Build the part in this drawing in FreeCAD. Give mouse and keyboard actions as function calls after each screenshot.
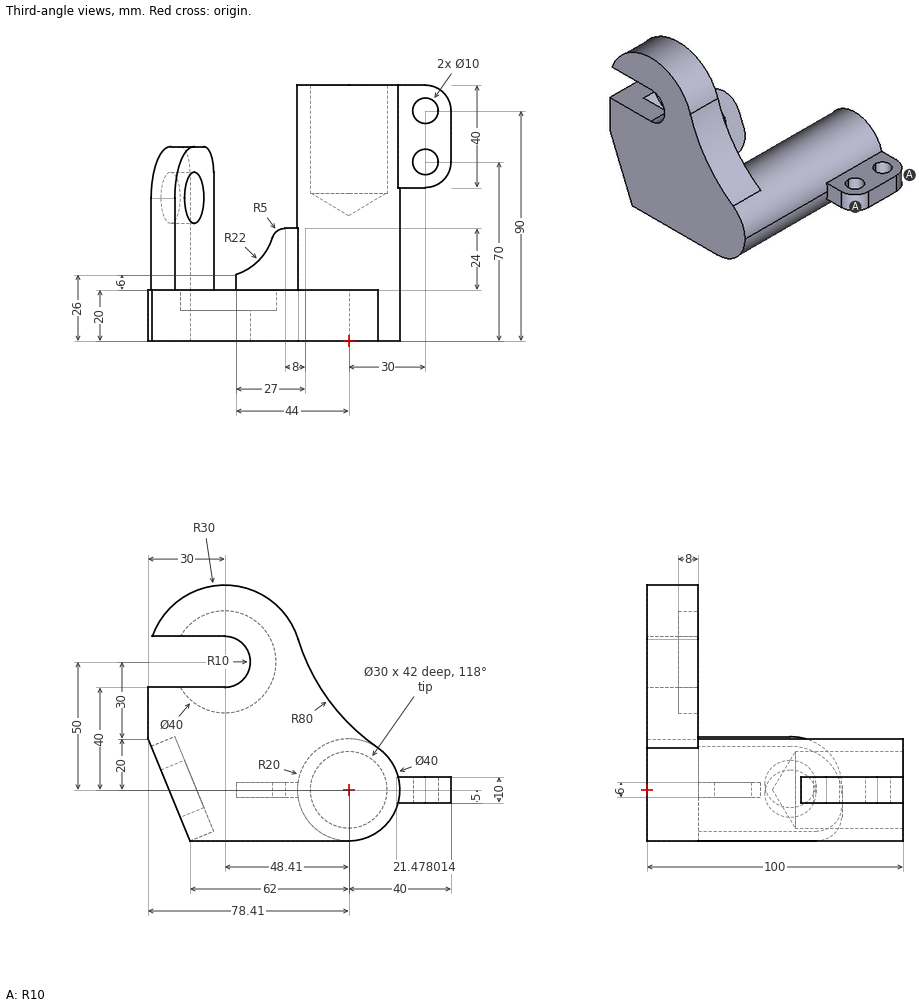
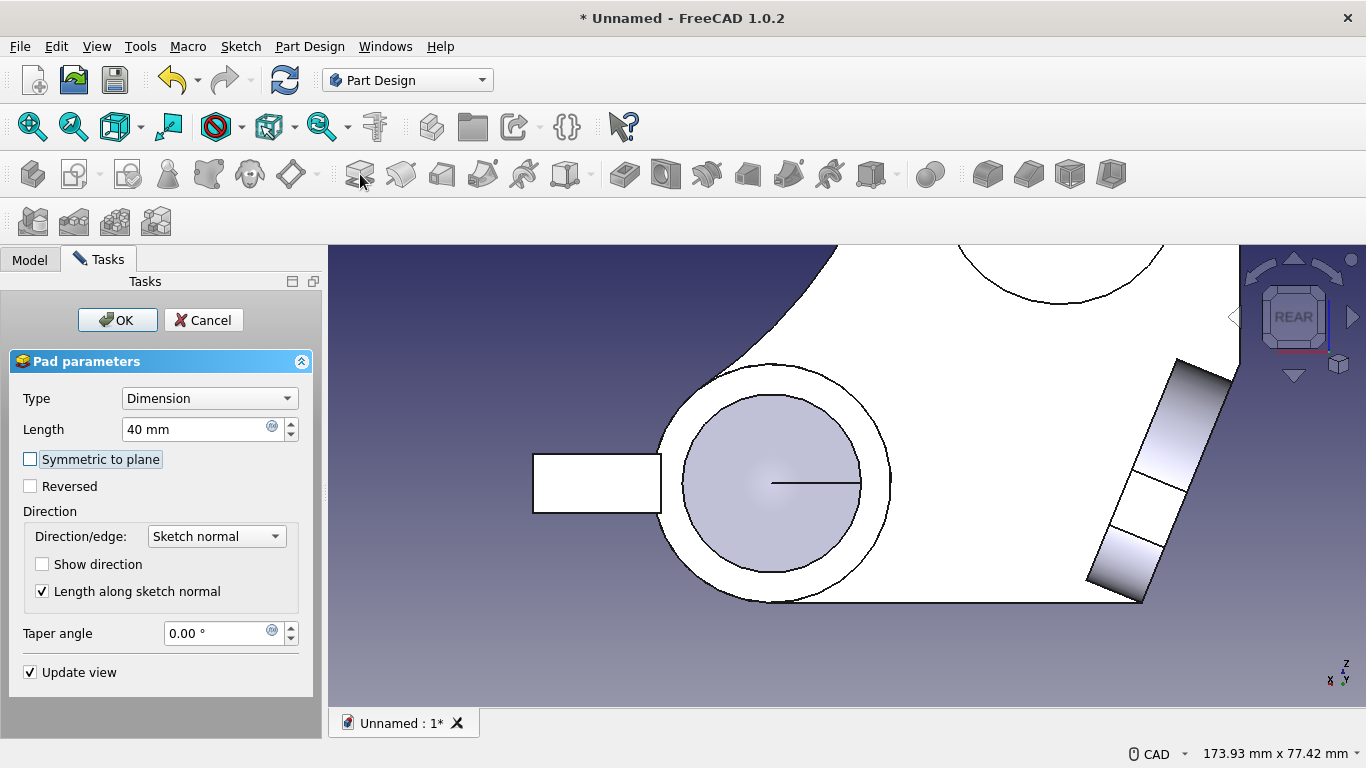
click(31, 486)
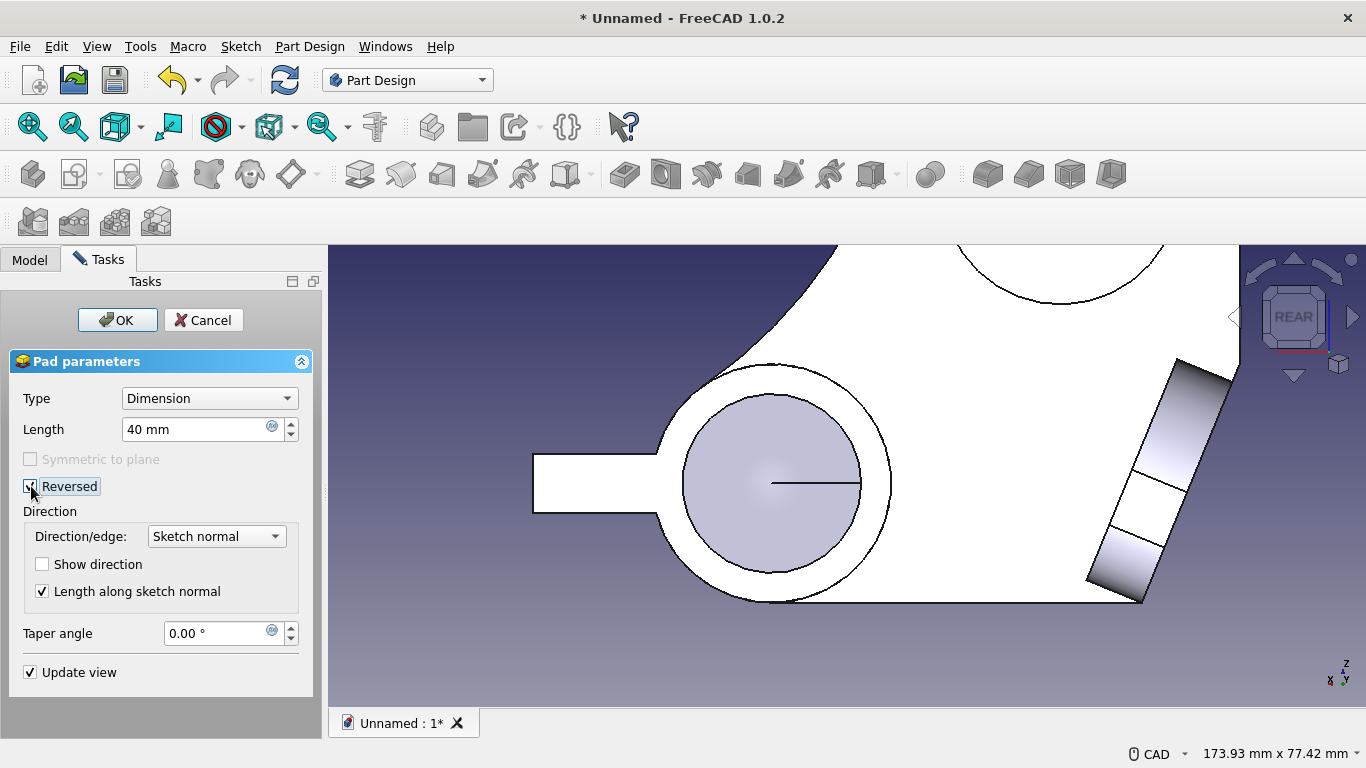
click(118, 320)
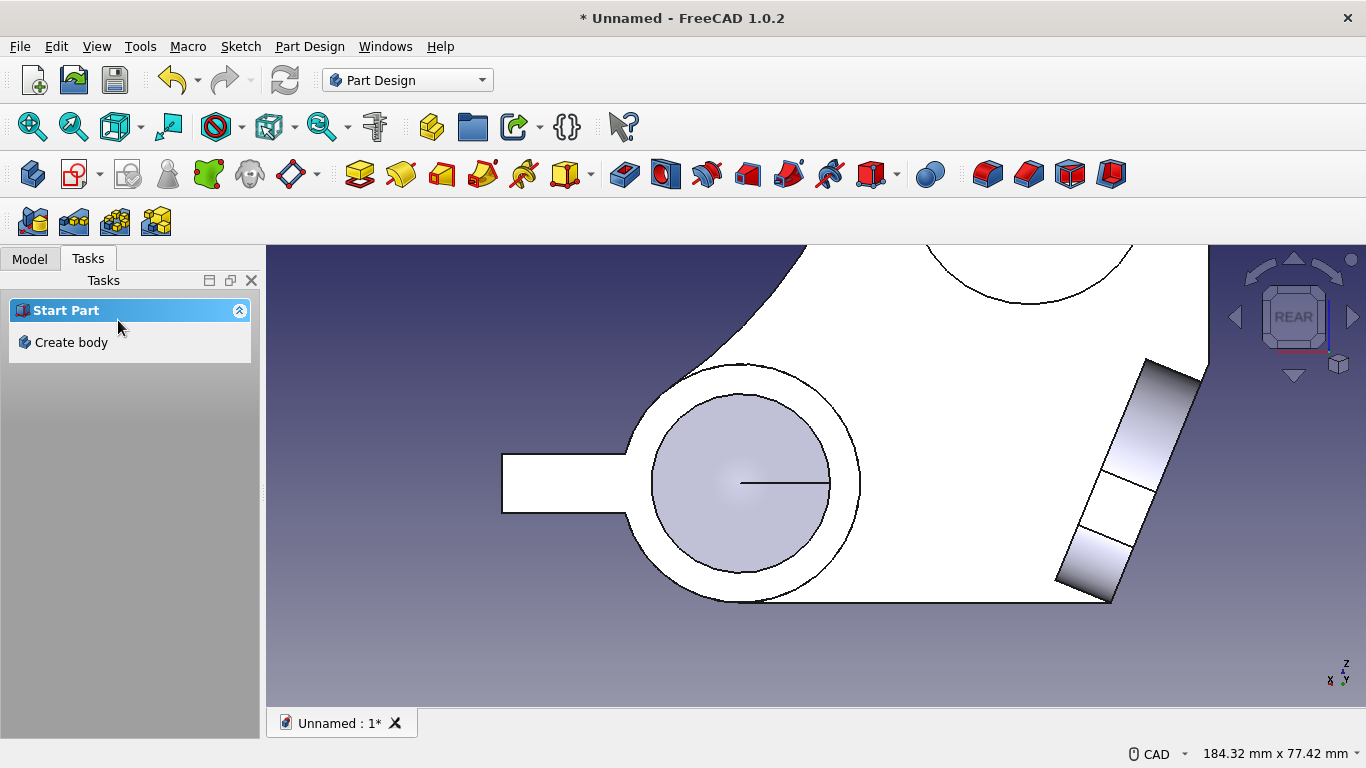
key(v)
key(f)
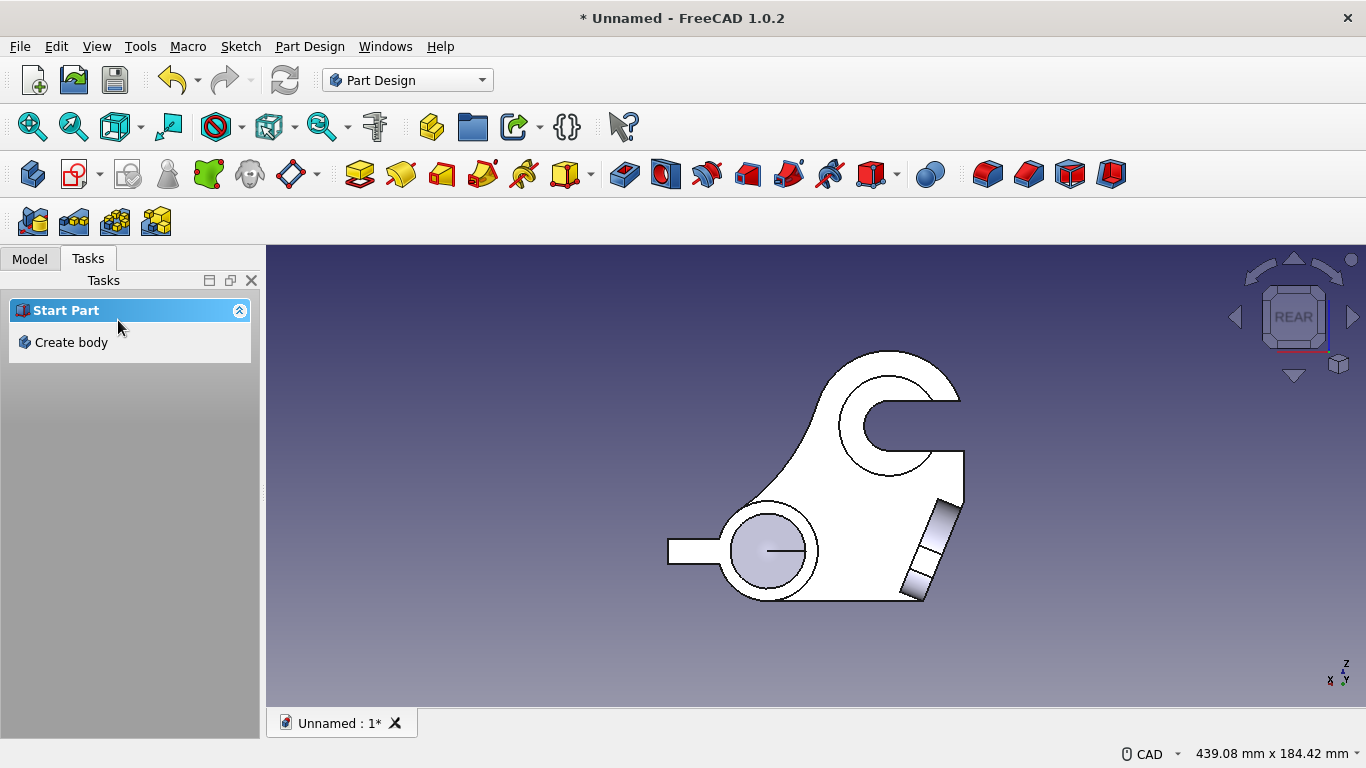
key(0)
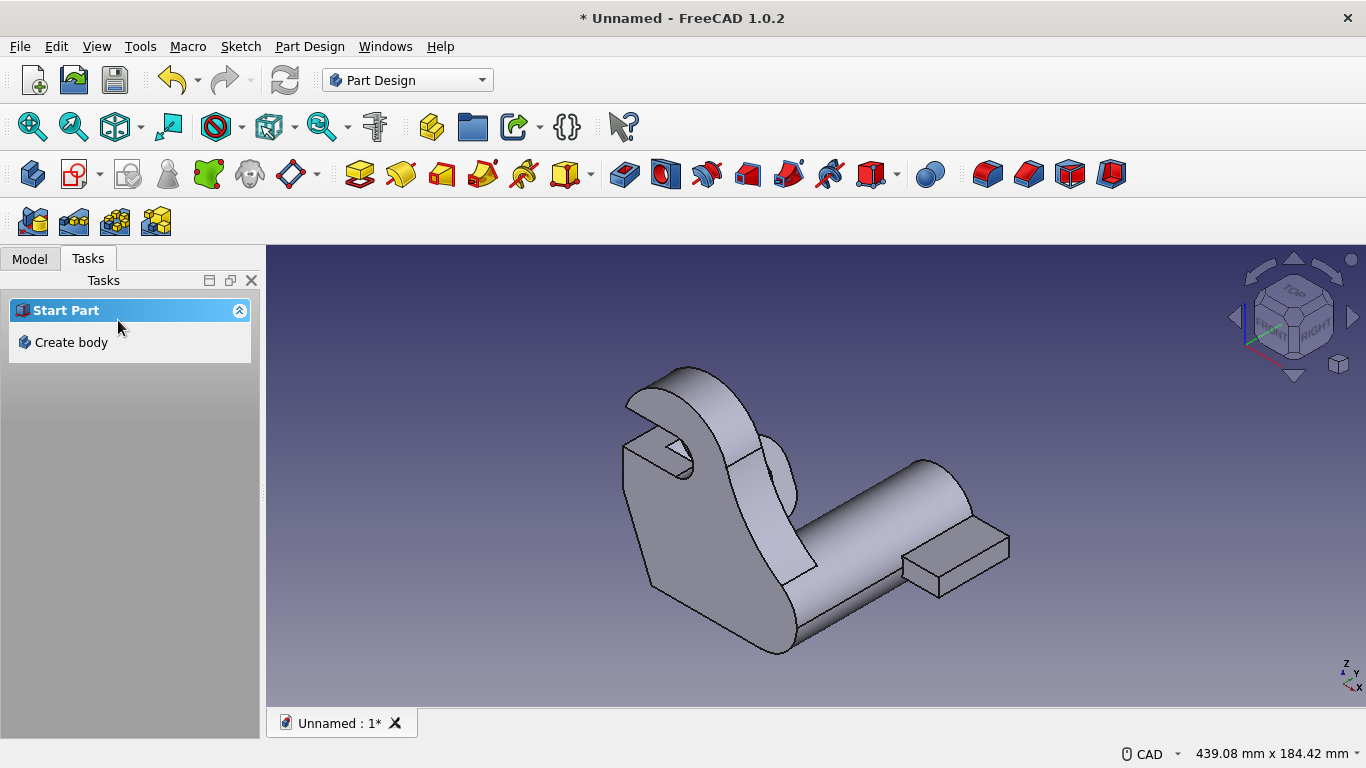
click(939, 587)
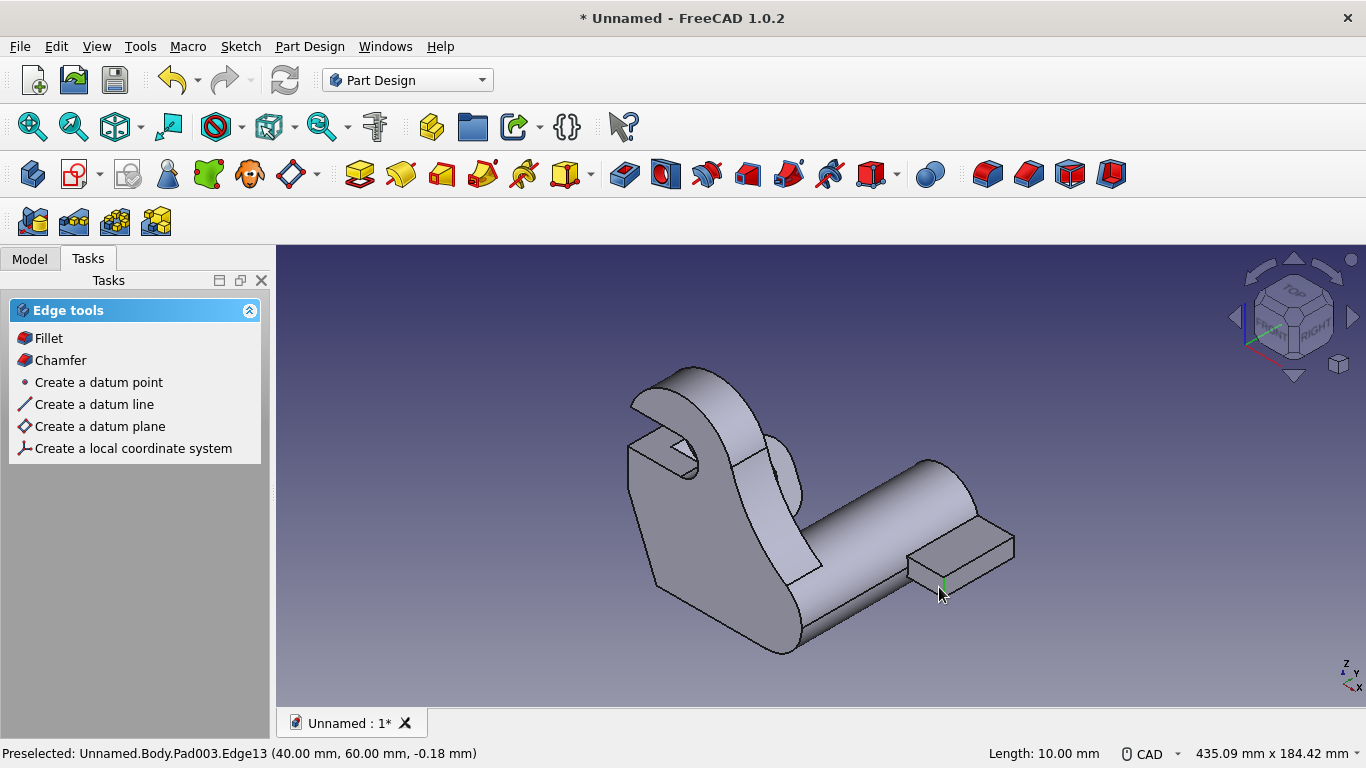
key(2)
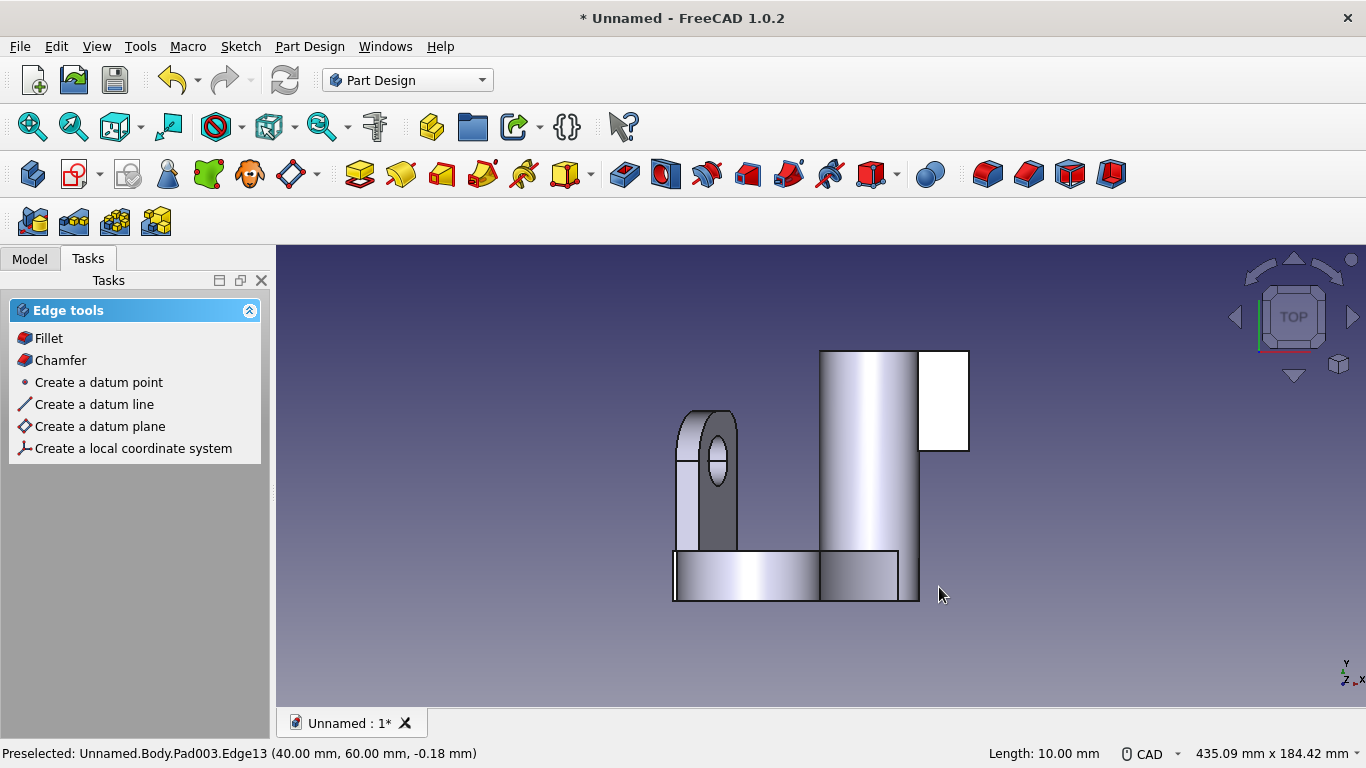
key(1)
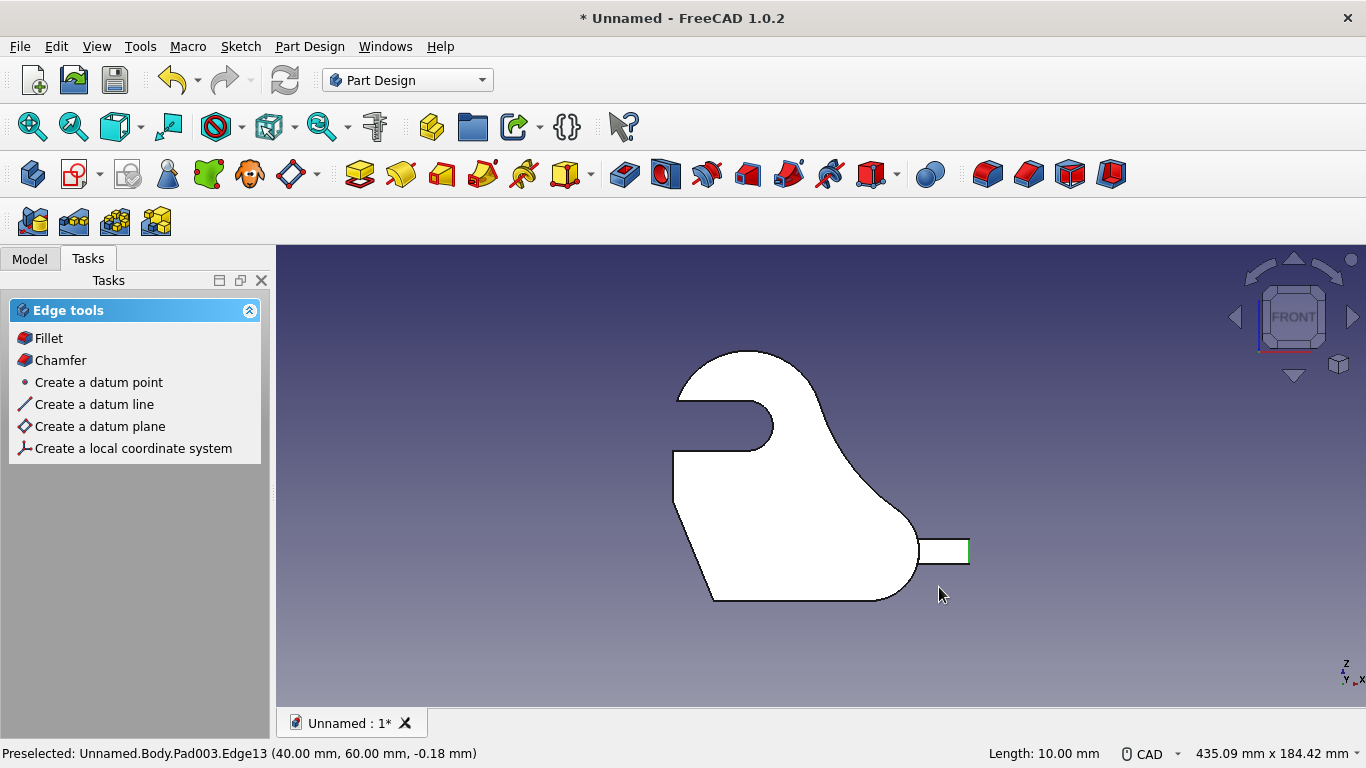
key(3)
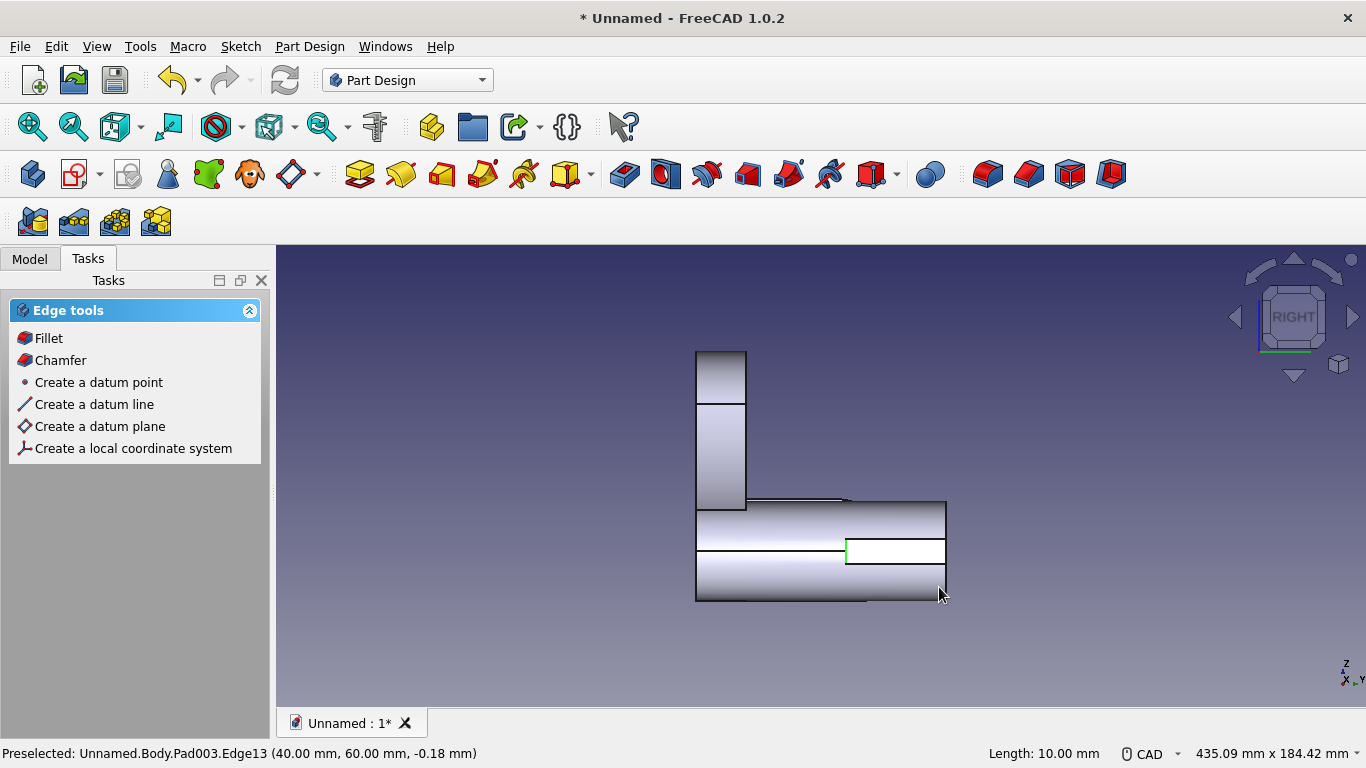
click(946, 550, ctrl)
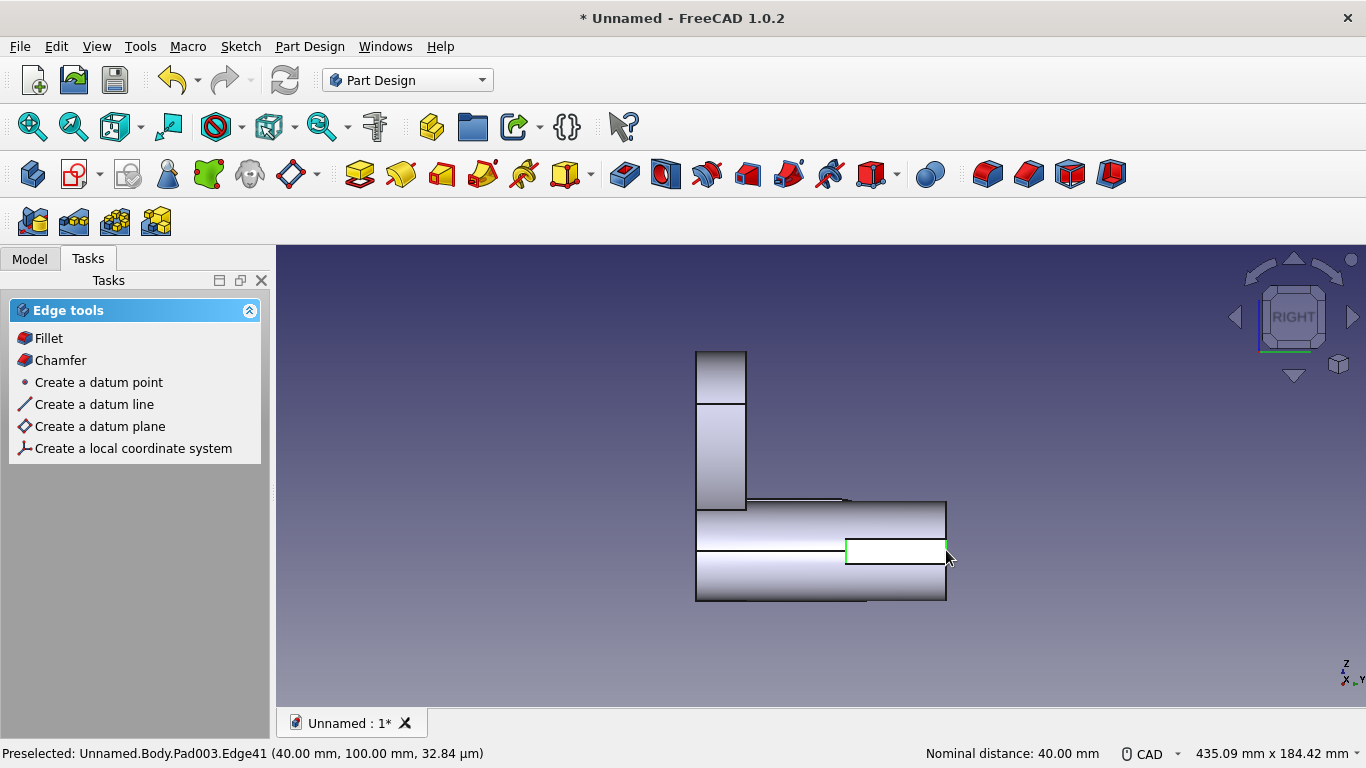
click(988, 174)